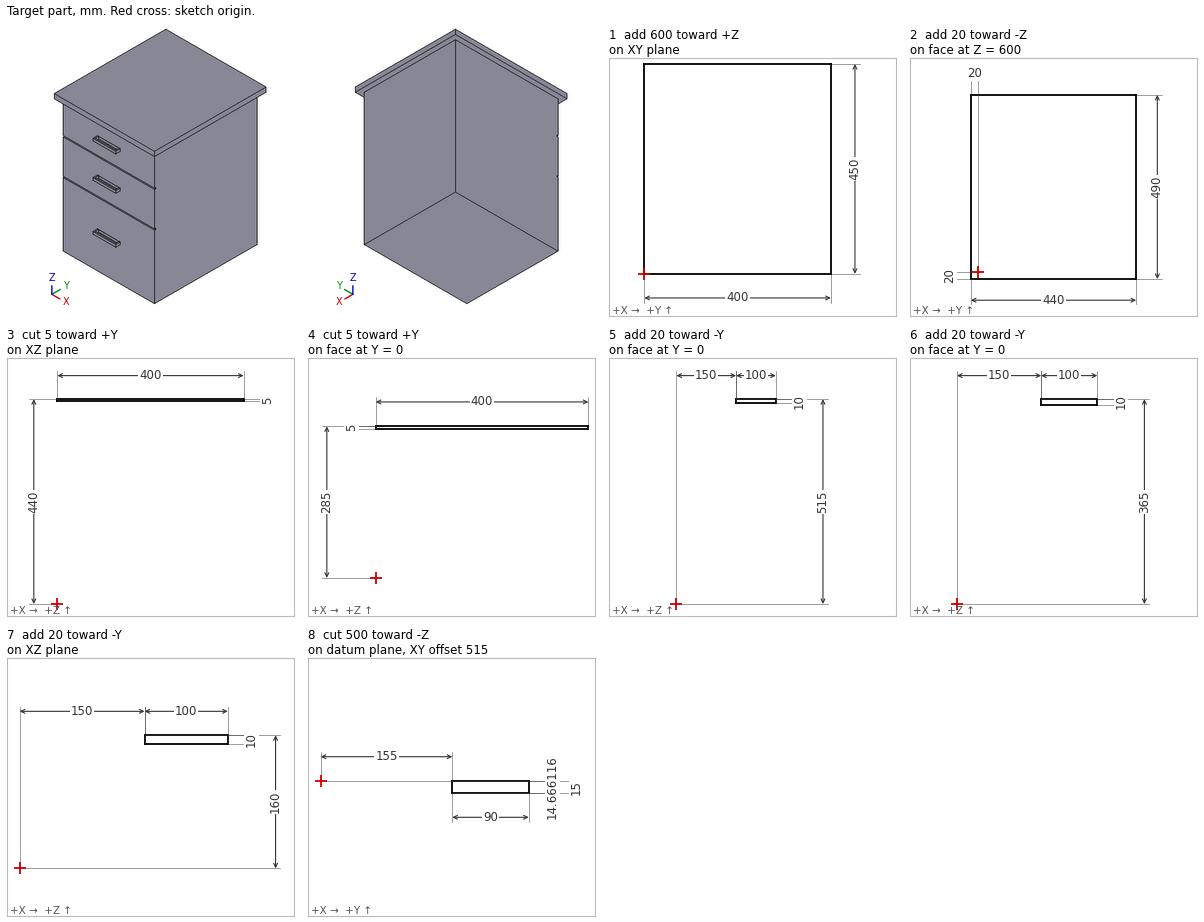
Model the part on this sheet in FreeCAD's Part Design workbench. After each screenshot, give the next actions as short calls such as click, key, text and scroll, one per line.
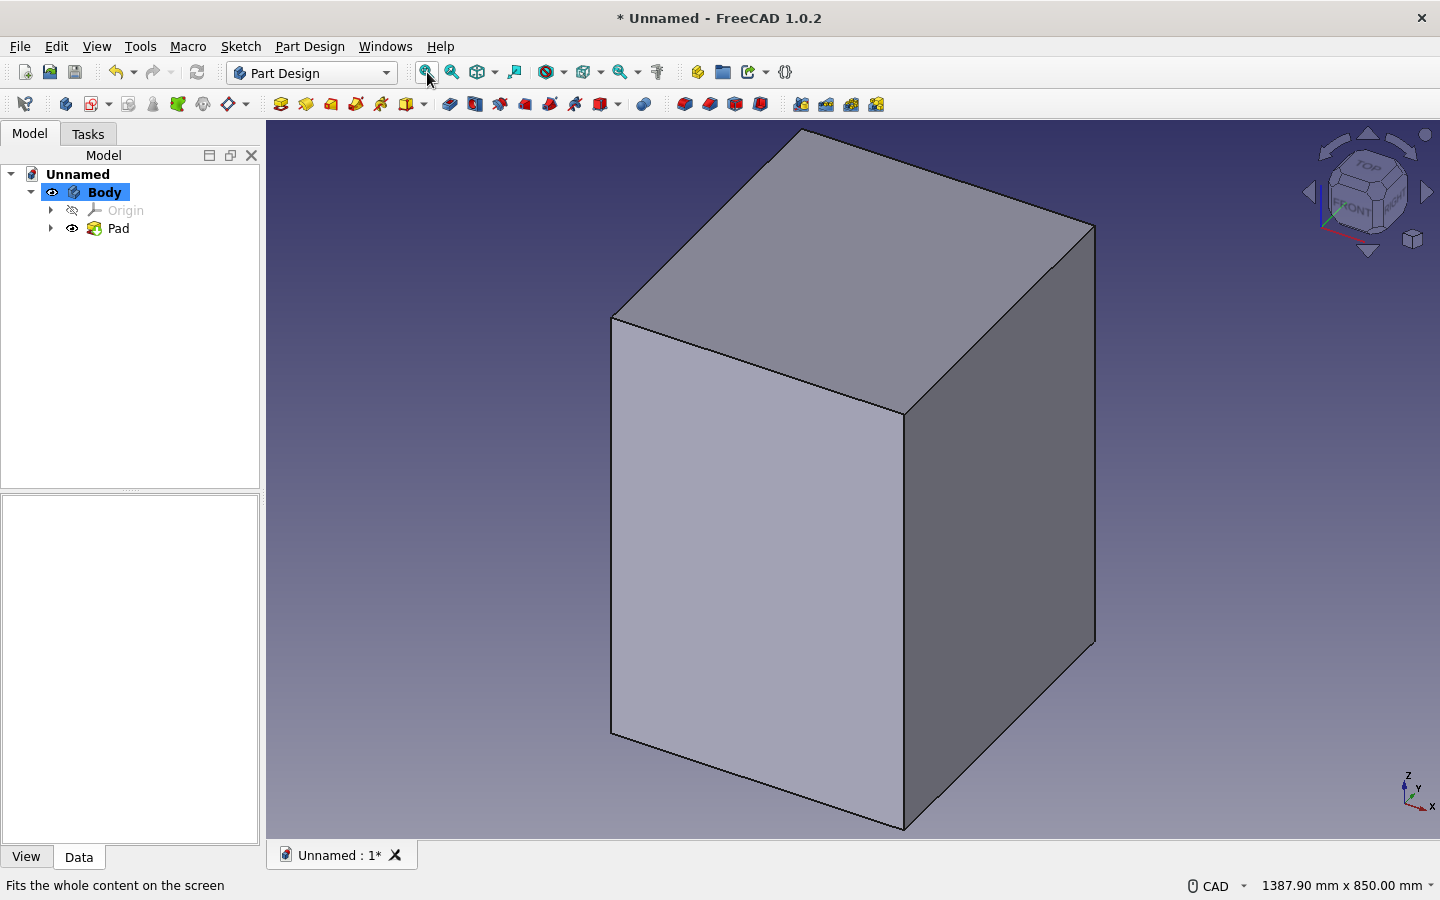
click(853, 271)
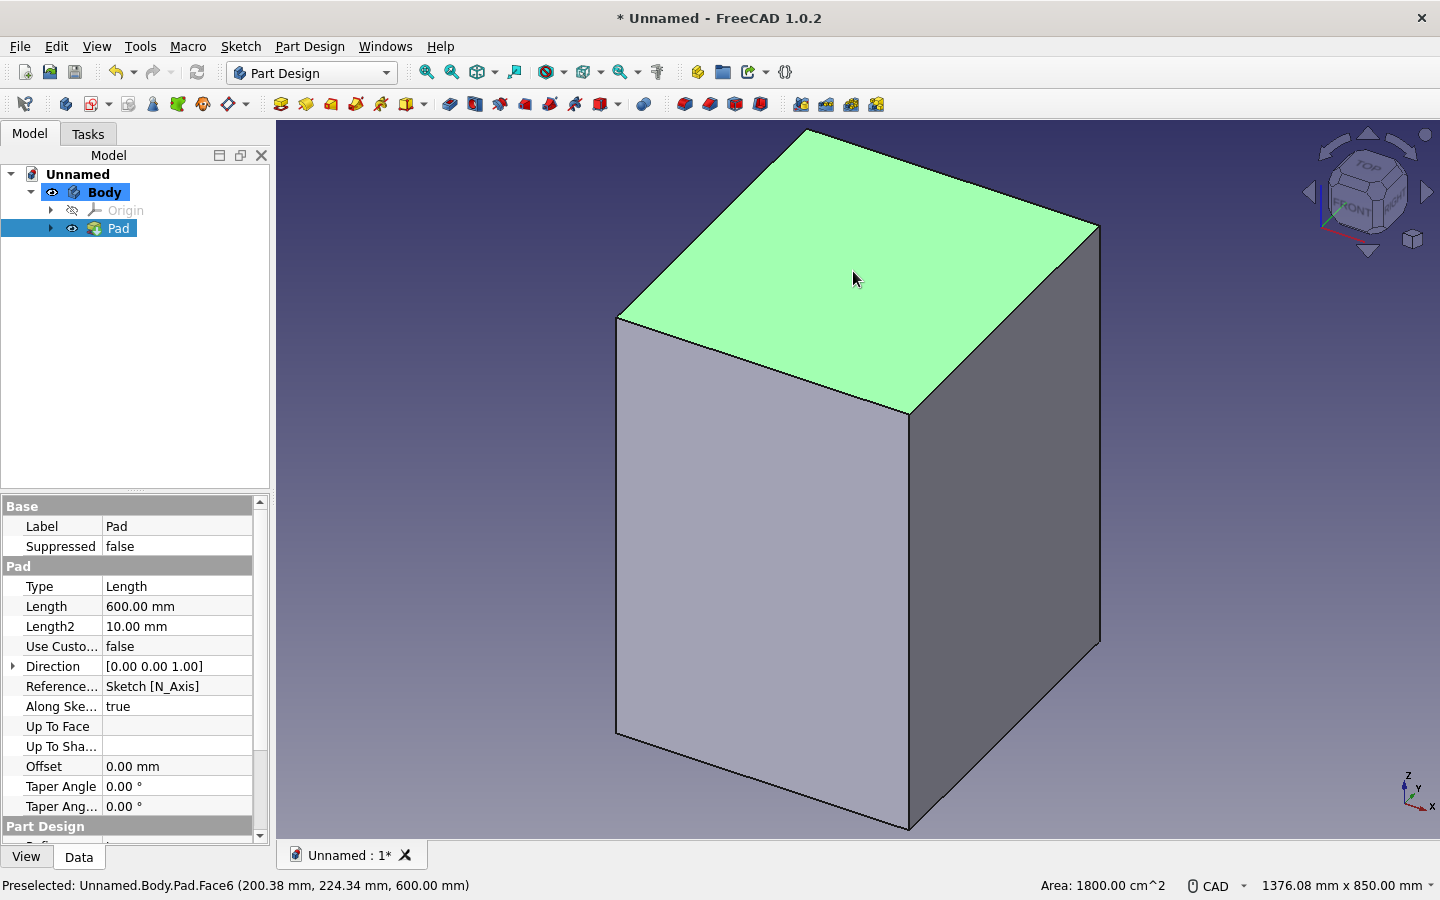
click(90, 104)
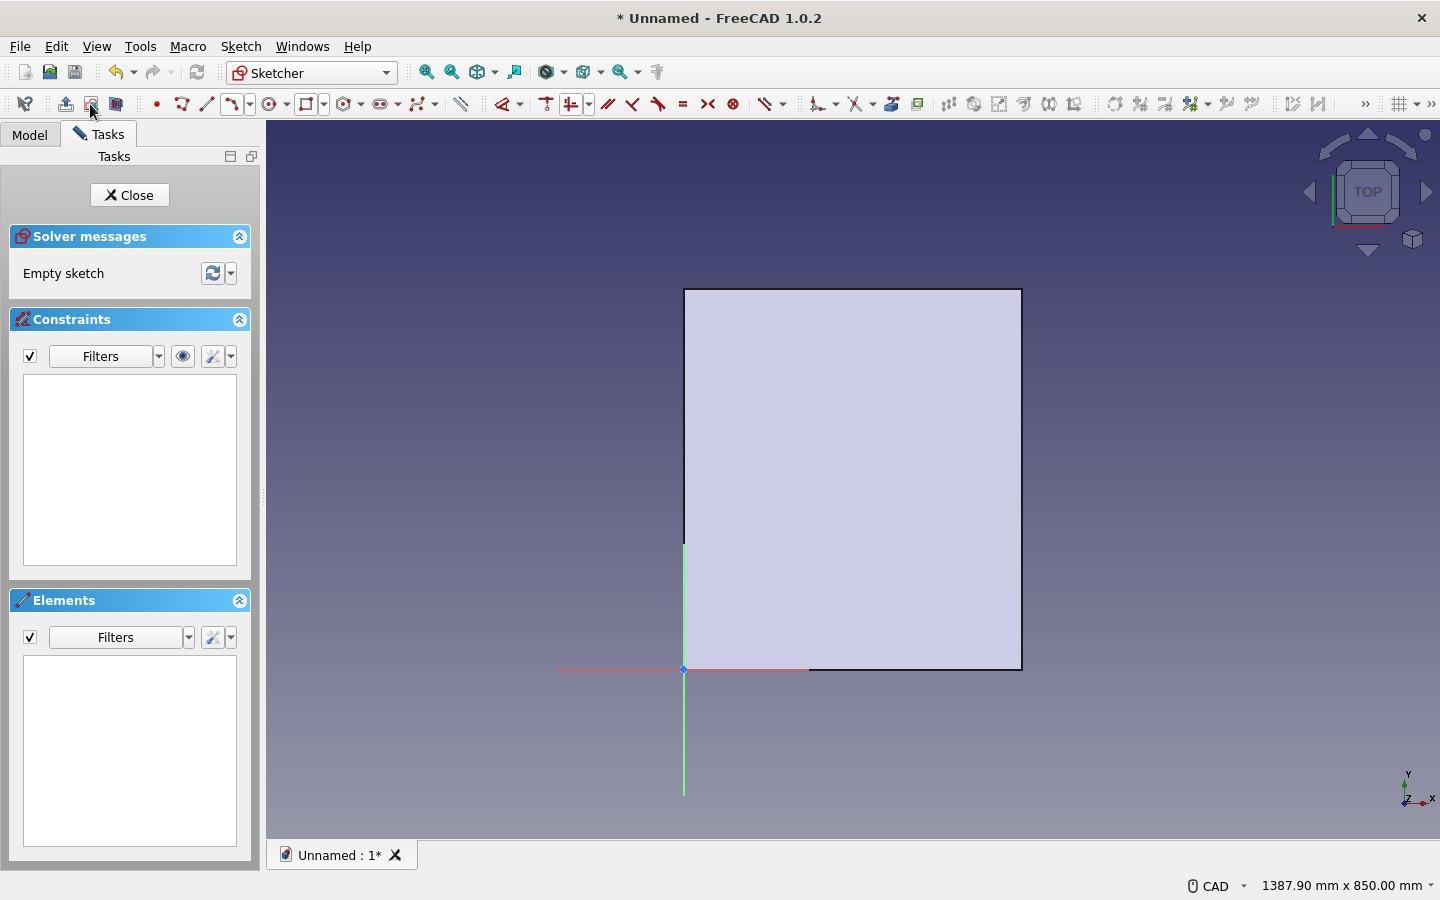
key(g)
key(r)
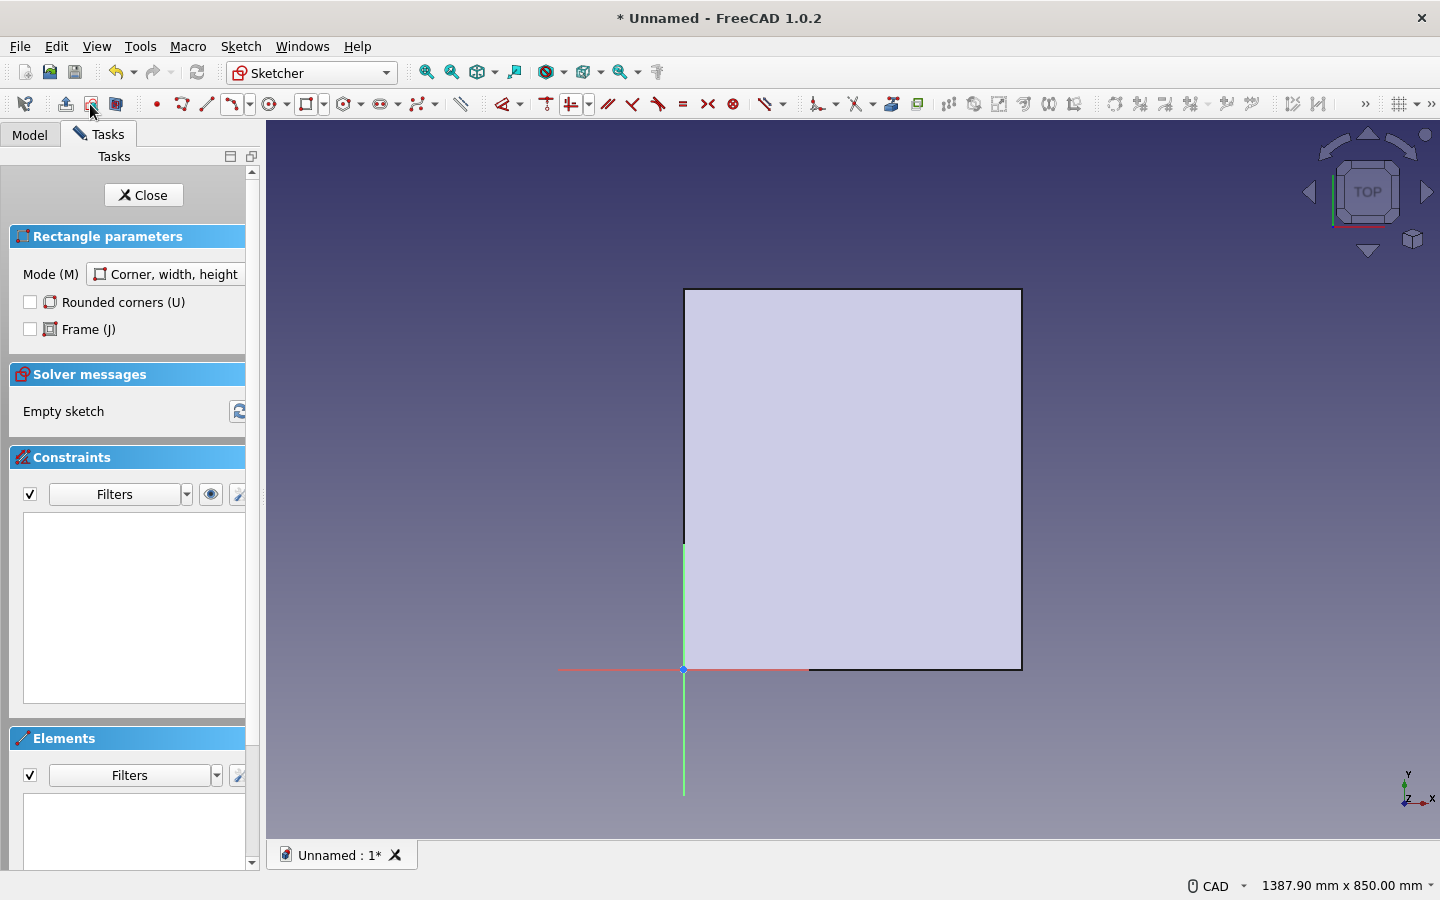
click(667, 272)
move(1039, 687)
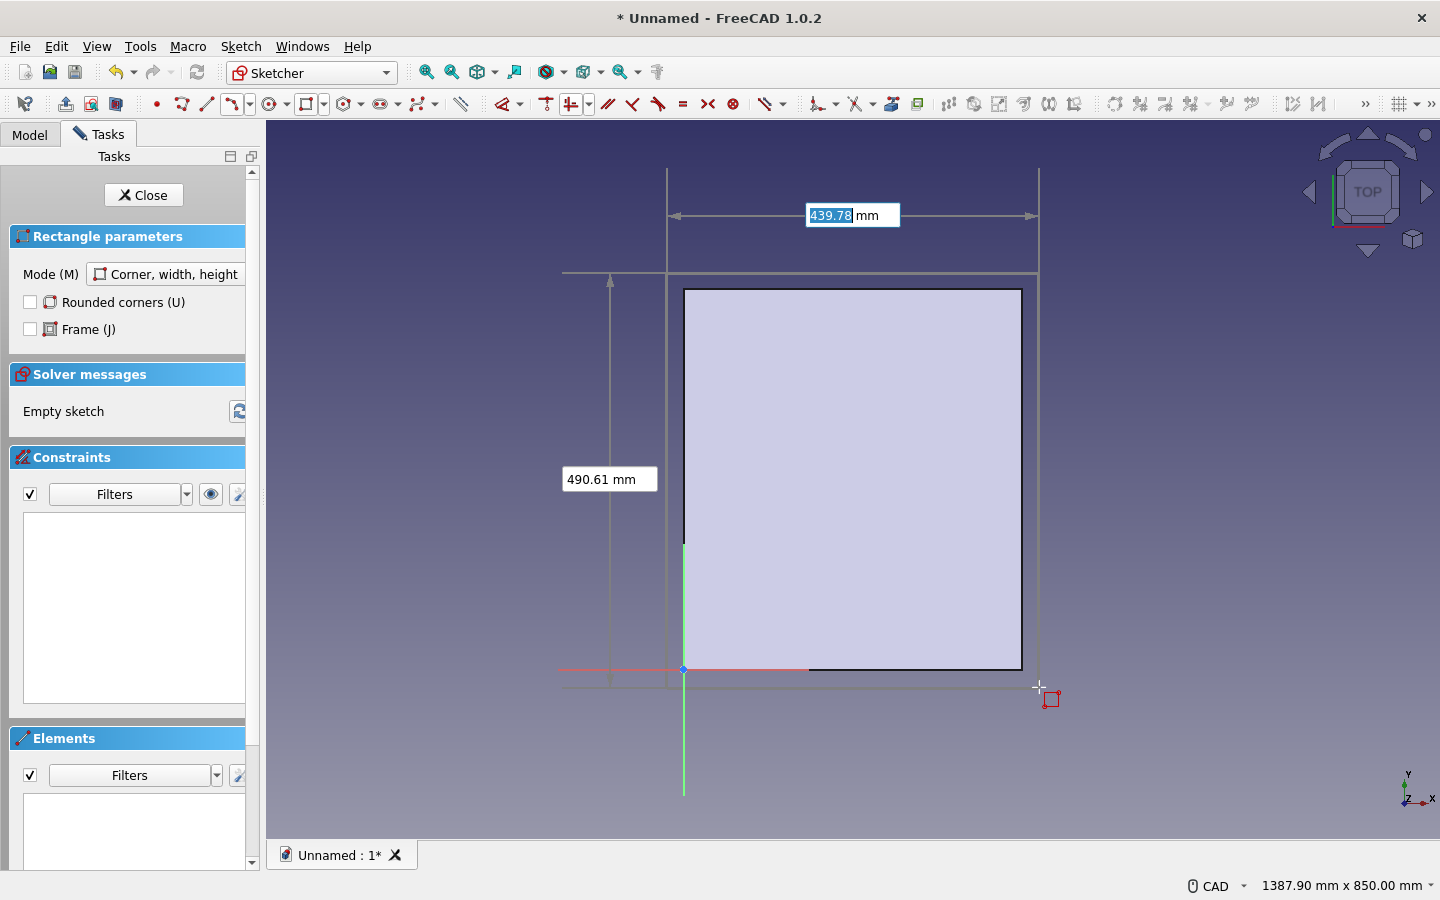
text(440)
key(Tab)
text(490)
key(Return)
key(Escape)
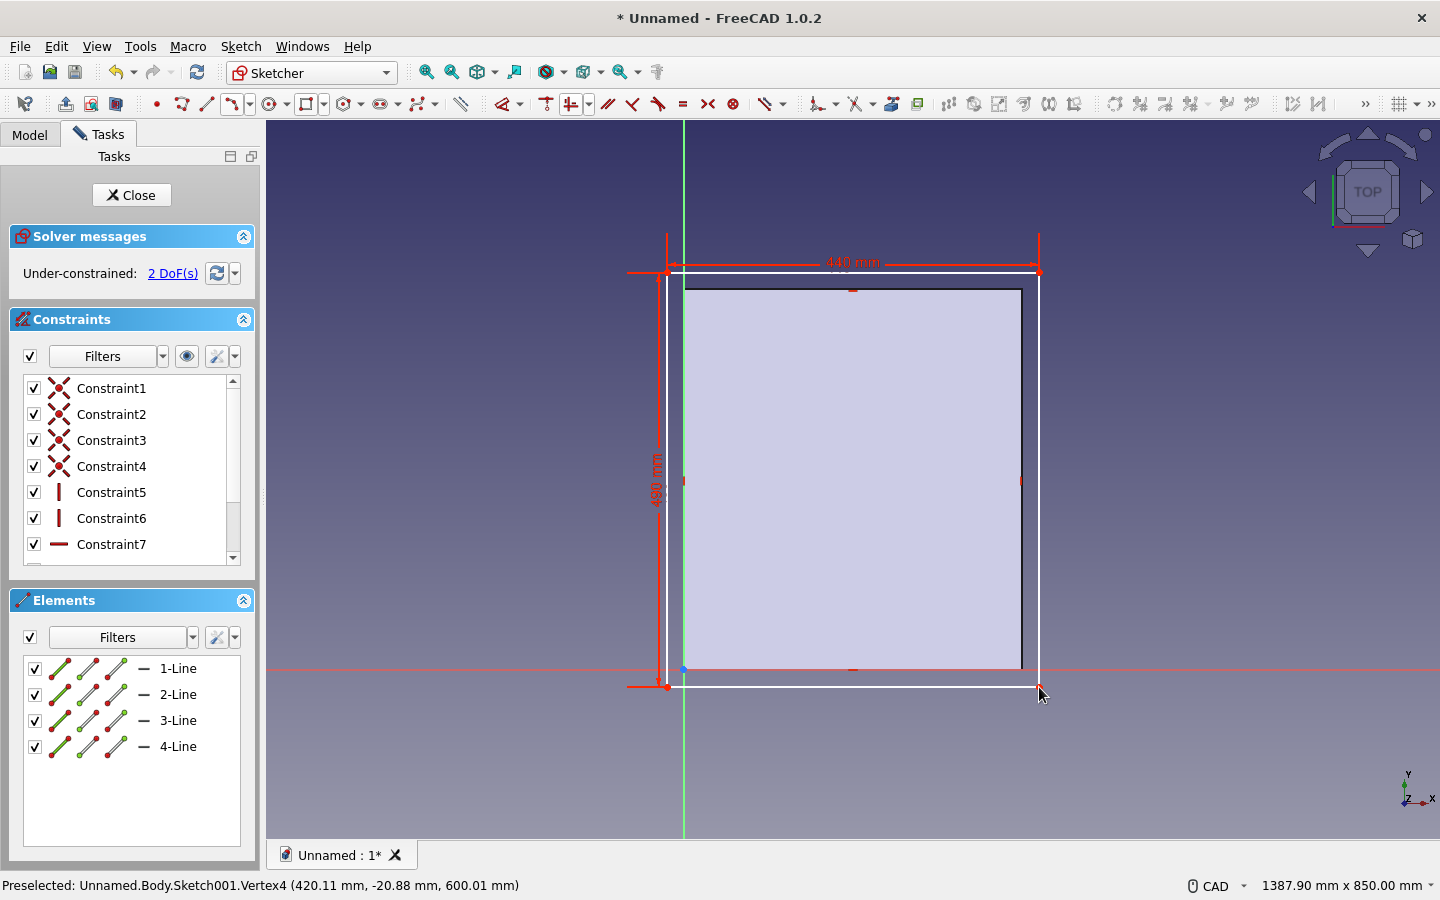
click(502, 104)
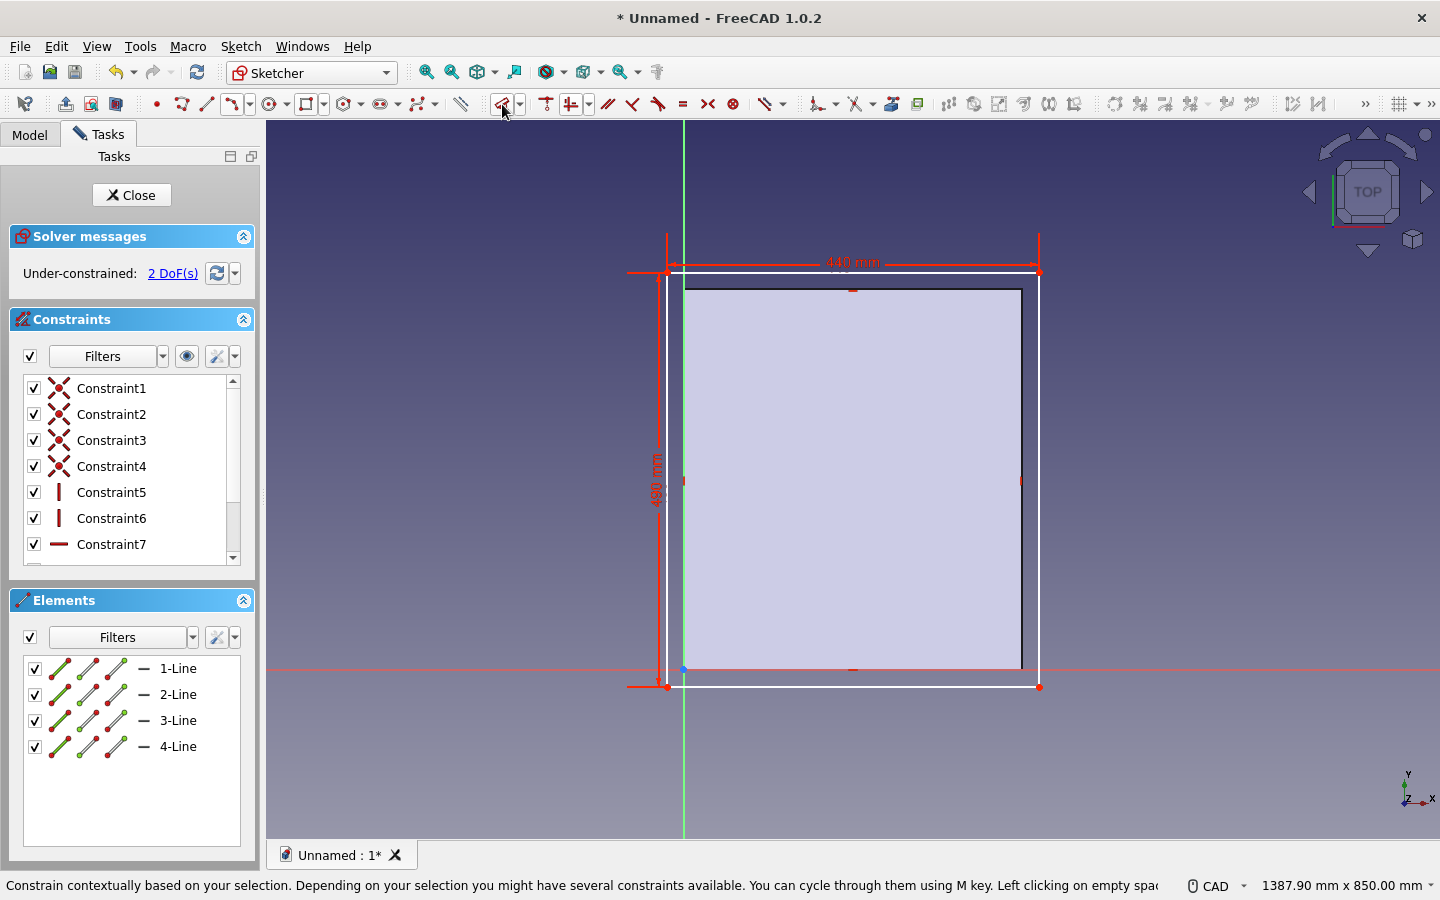
scroll(667, 273, up, 5)